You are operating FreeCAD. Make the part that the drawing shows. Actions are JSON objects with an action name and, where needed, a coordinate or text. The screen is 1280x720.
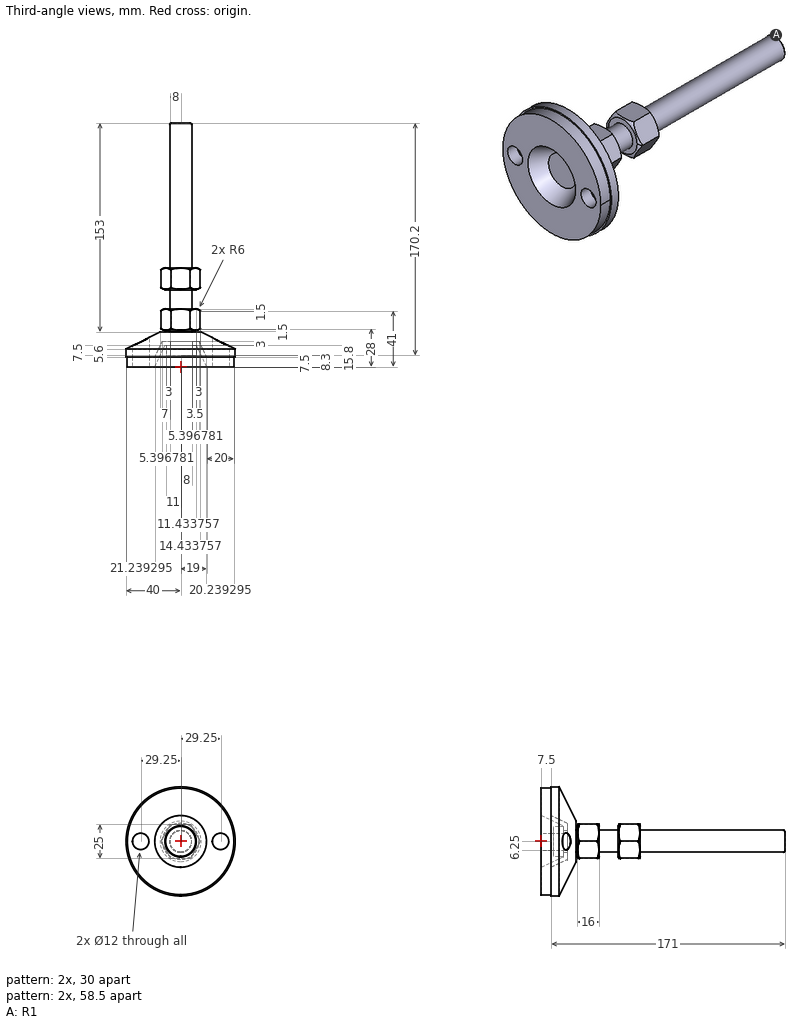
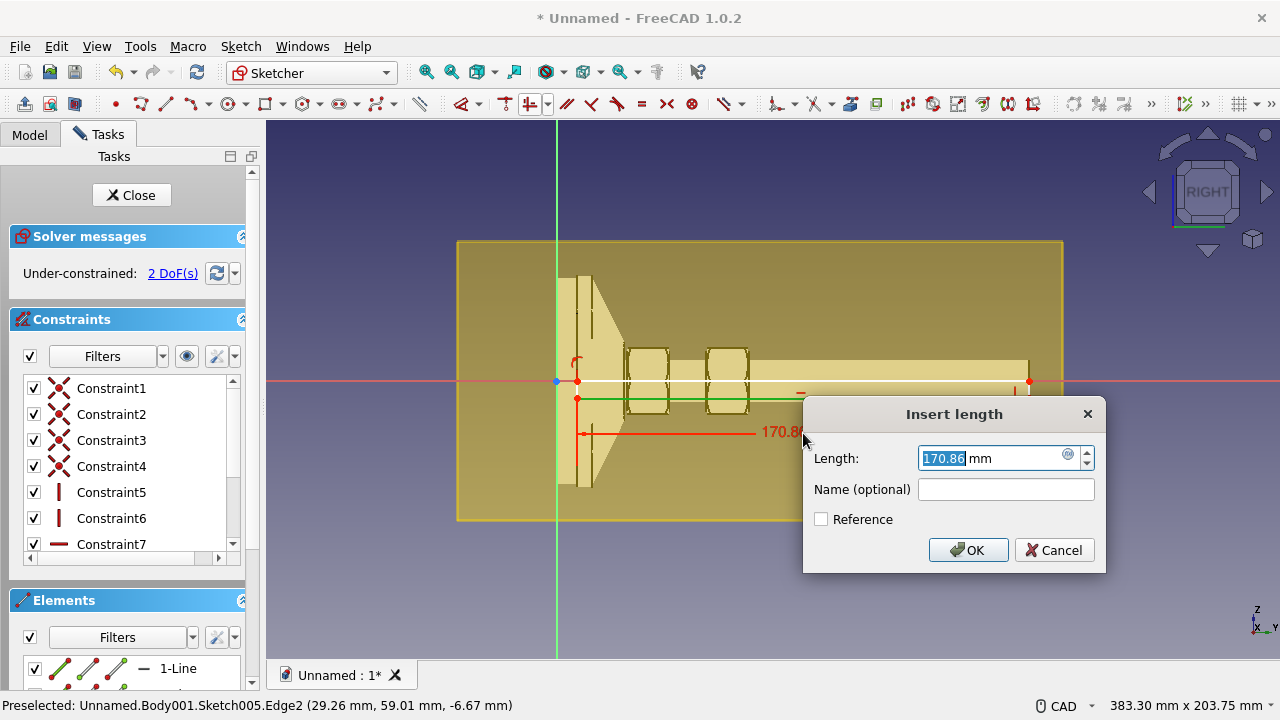
{"action": "type", "text": "171"}
{"action": "key", "text": "Return"}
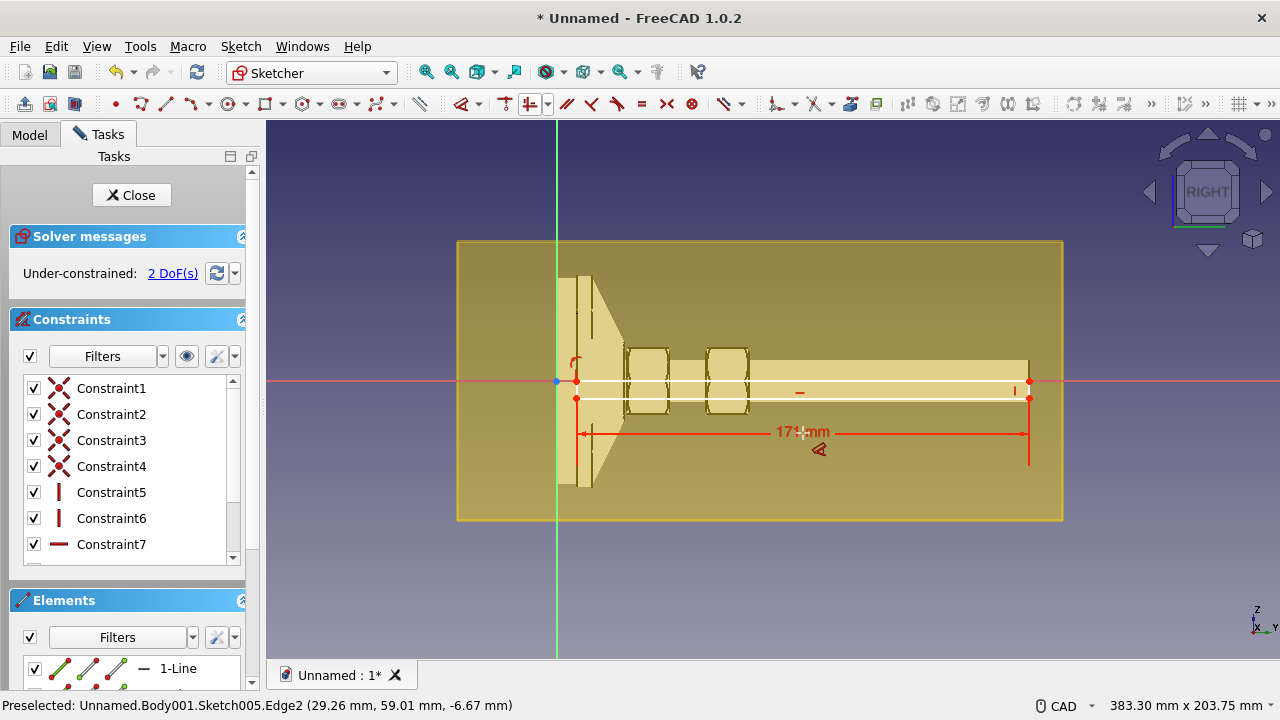
{"action": "scroll", "coordinate": [577, 390], "scroll_direction": "up", "scroll_amount": 5}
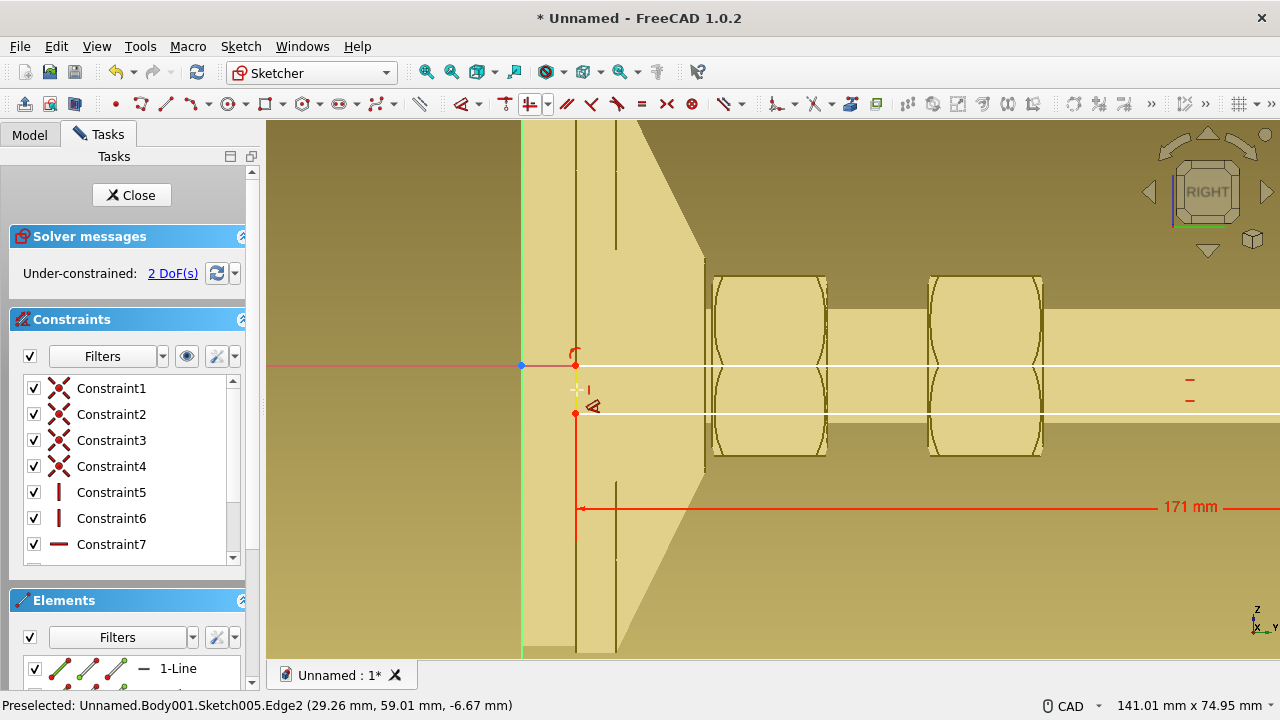
{"action": "left_click", "coordinate": [576, 390]}
{"action": "left_click", "coordinate": [542, 390]}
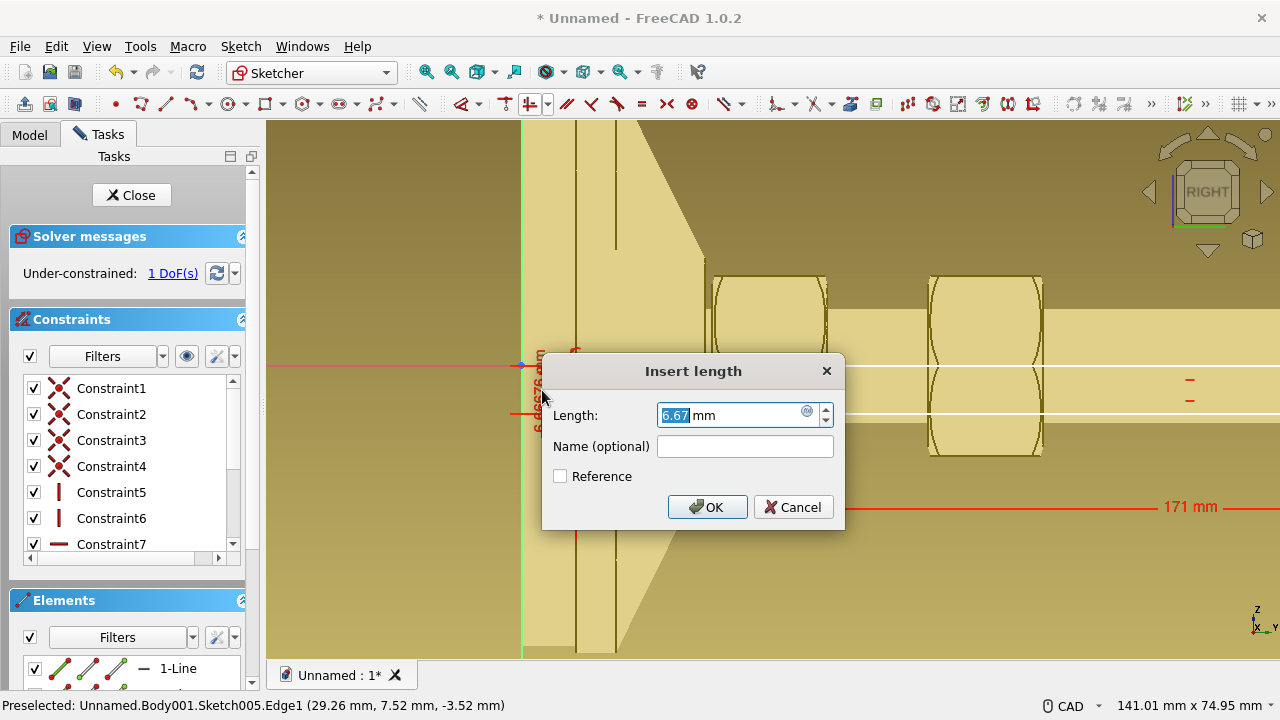
{"action": "type", "text": "6.25"}
{"action": "key", "text": "Return"}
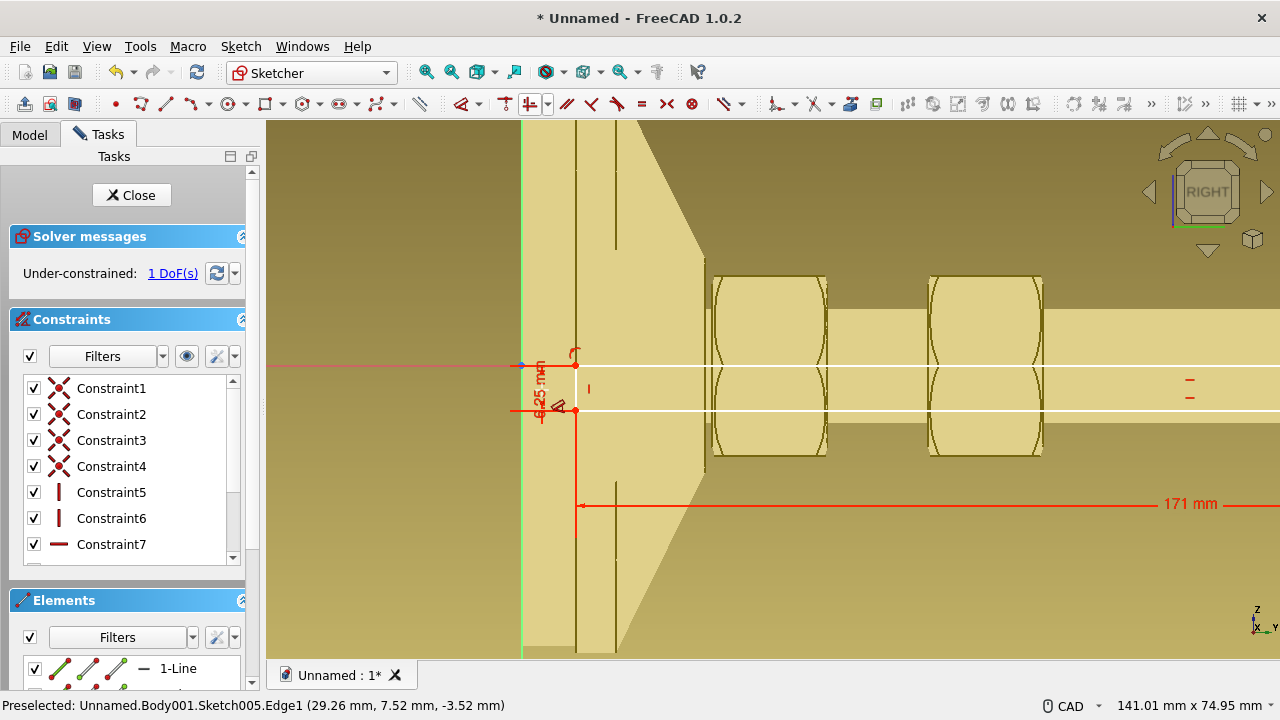
{"action": "left_click", "coordinate": [576, 366]}
{"action": "left_click", "coordinate": [549, 332]}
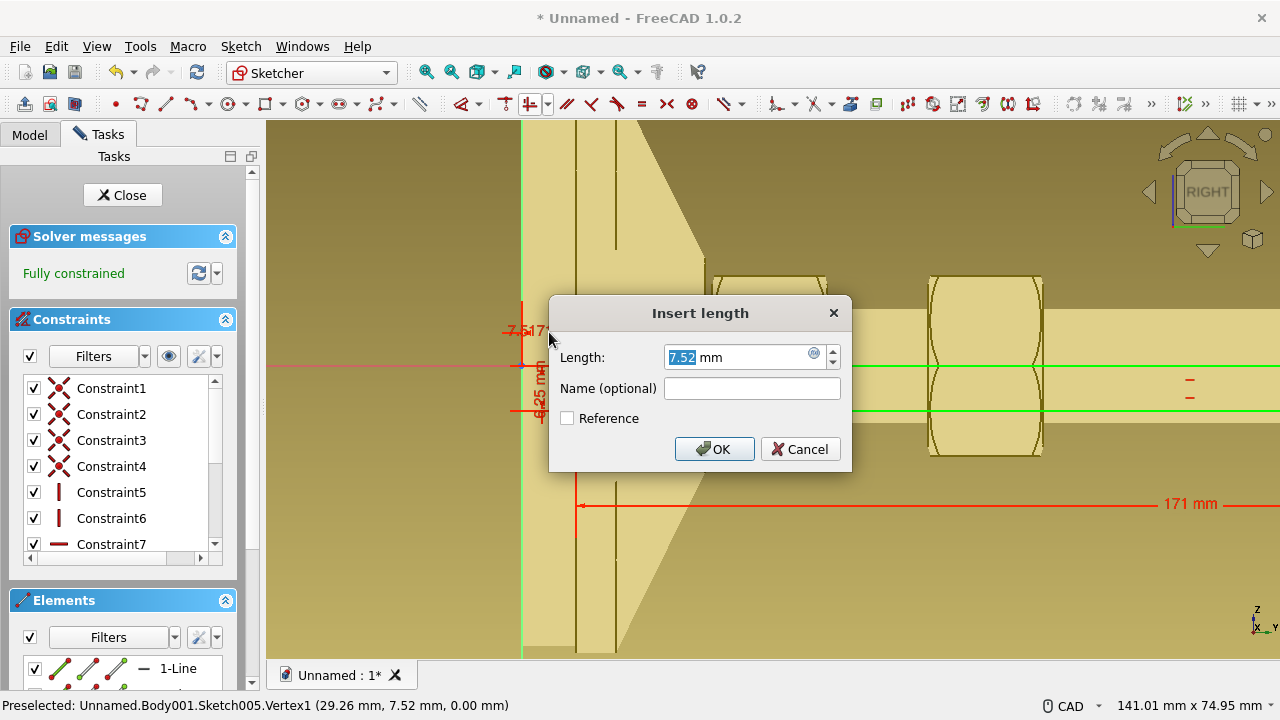
{"action": "type", "text": "7.5"}
{"action": "key", "text": "Return"}
{"action": "key", "text": "Escape"}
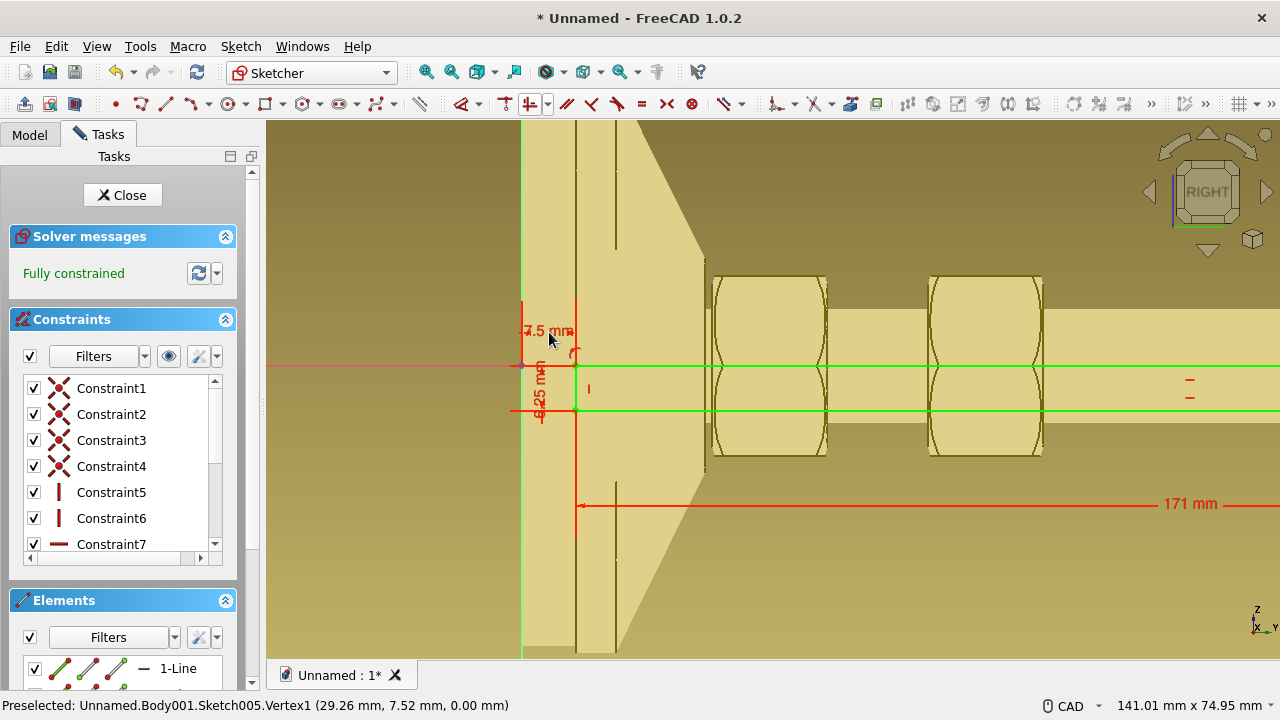
{"action": "left_click", "coordinate": [123, 195]}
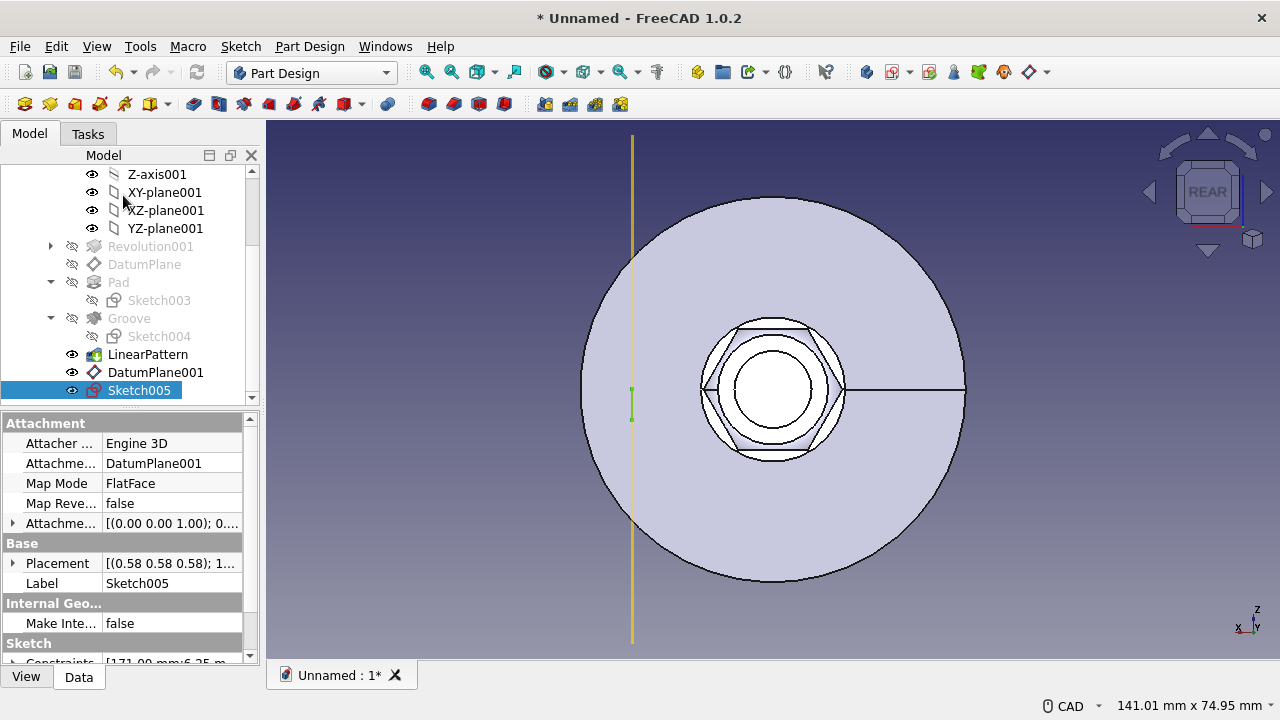
{"action": "left_click", "coordinate": [244, 104]}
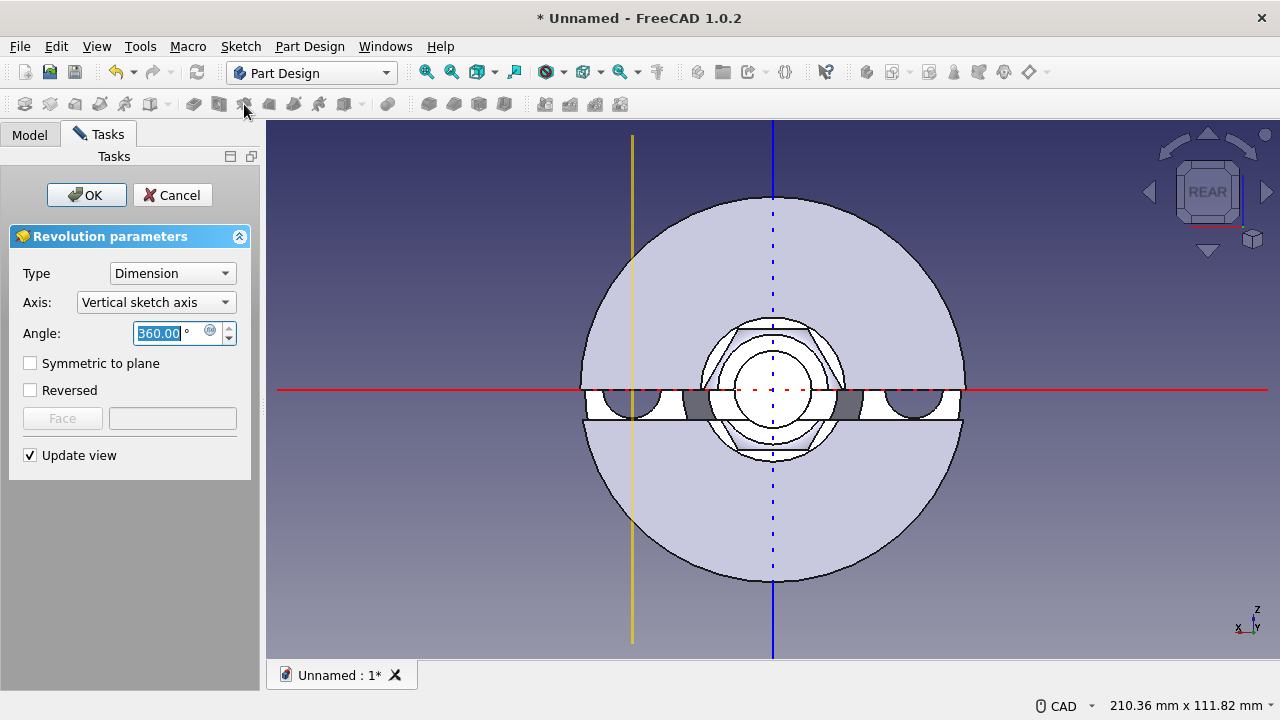
{"action": "left_click", "coordinate": [157, 302]}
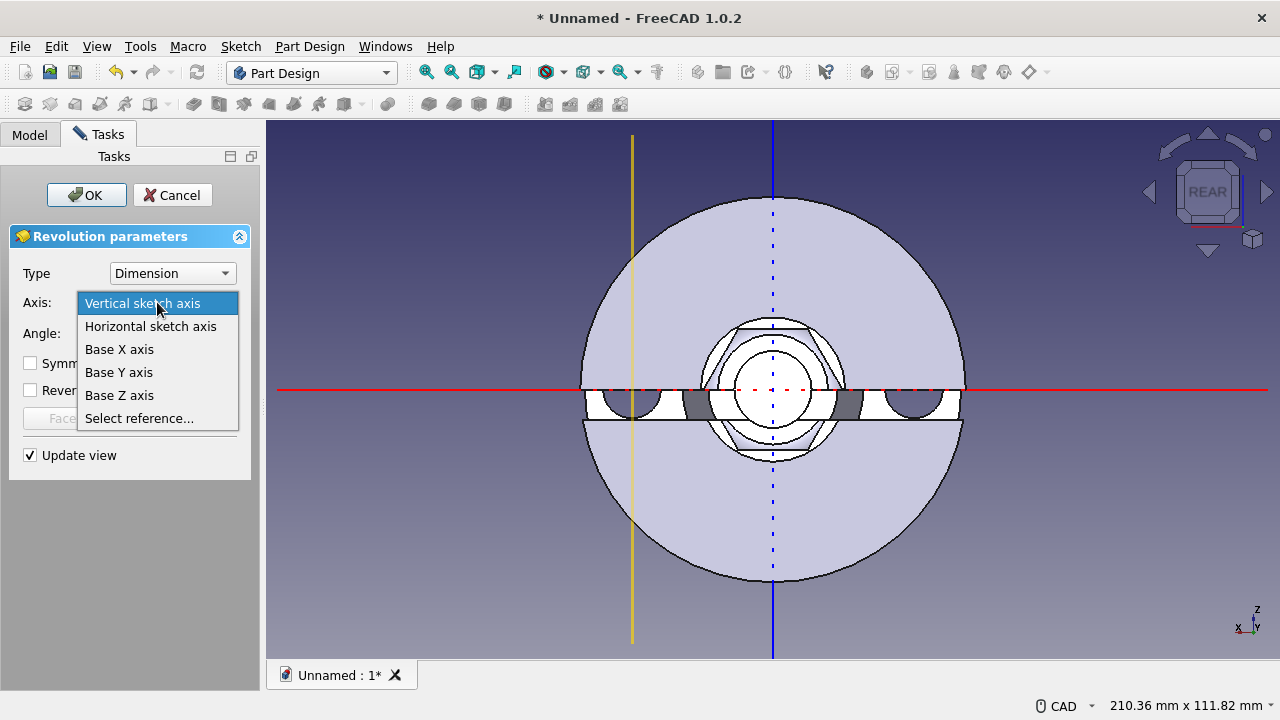
{"action": "left_click", "coordinate": [156, 326]}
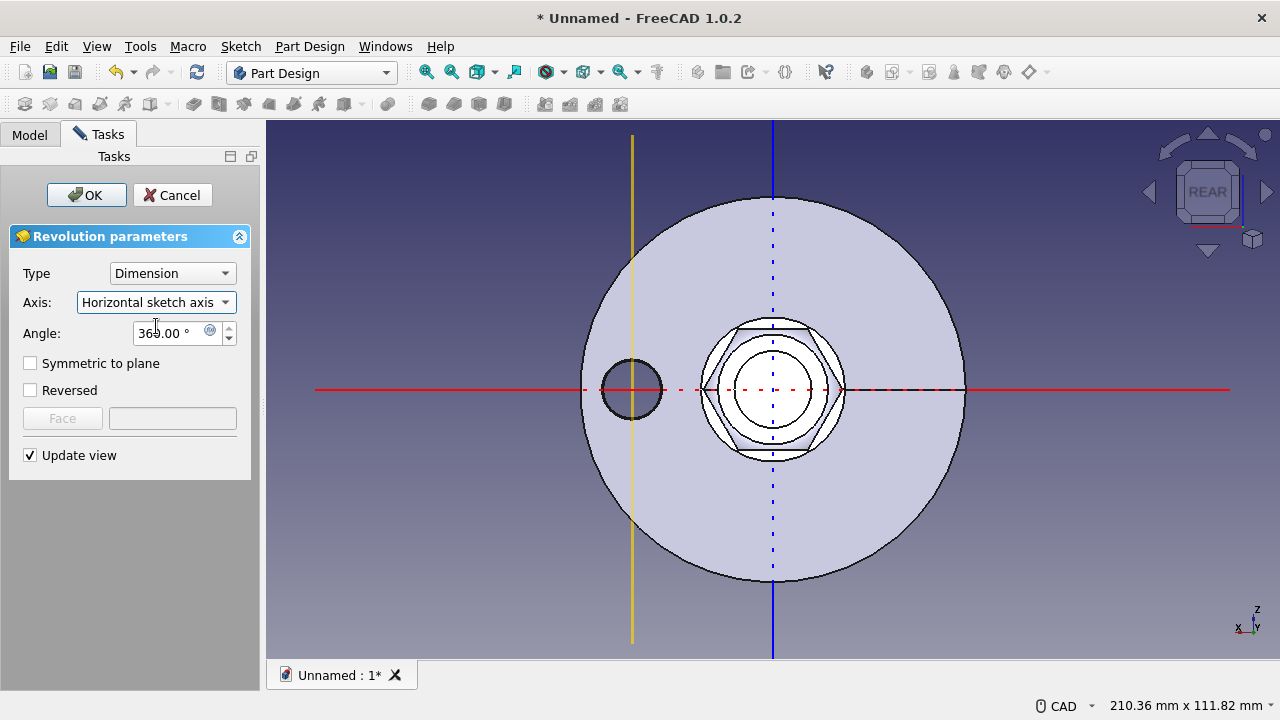
{"action": "left_click", "coordinate": [87, 195]}